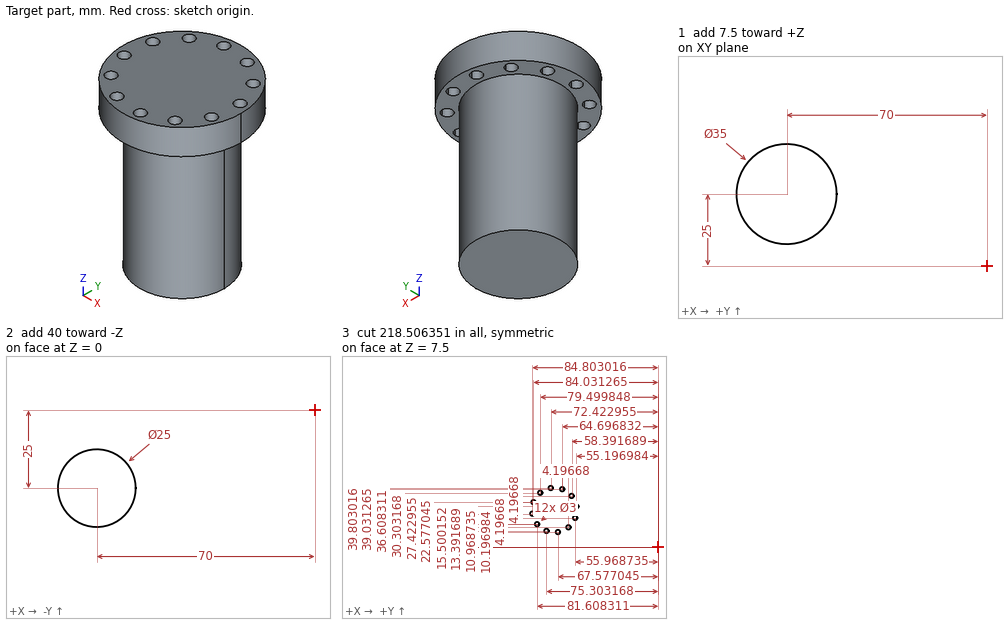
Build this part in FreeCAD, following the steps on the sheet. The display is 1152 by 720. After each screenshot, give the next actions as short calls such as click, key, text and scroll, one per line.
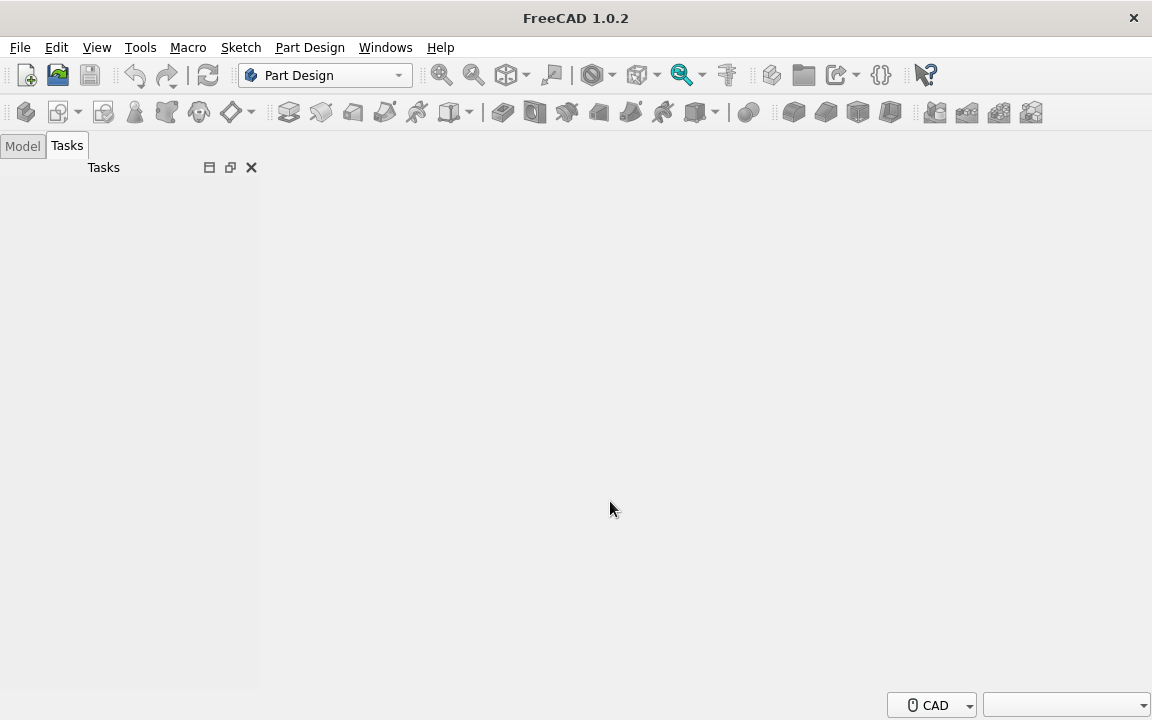
key(ctrl+n)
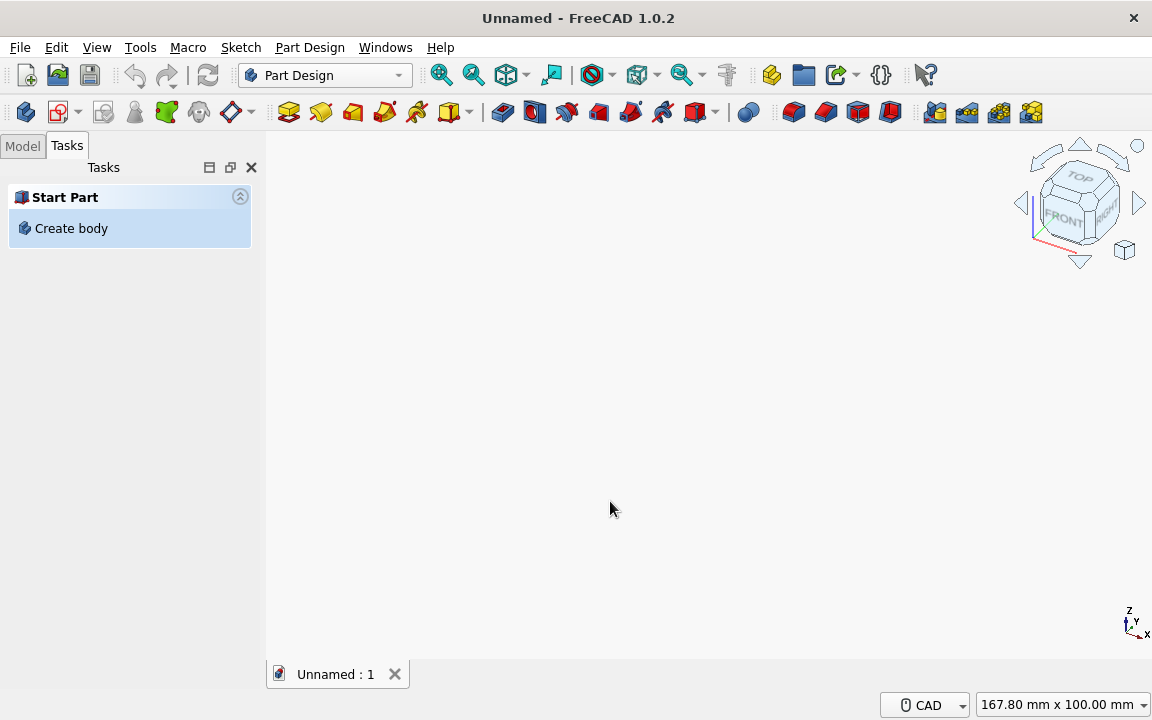
click(58, 112)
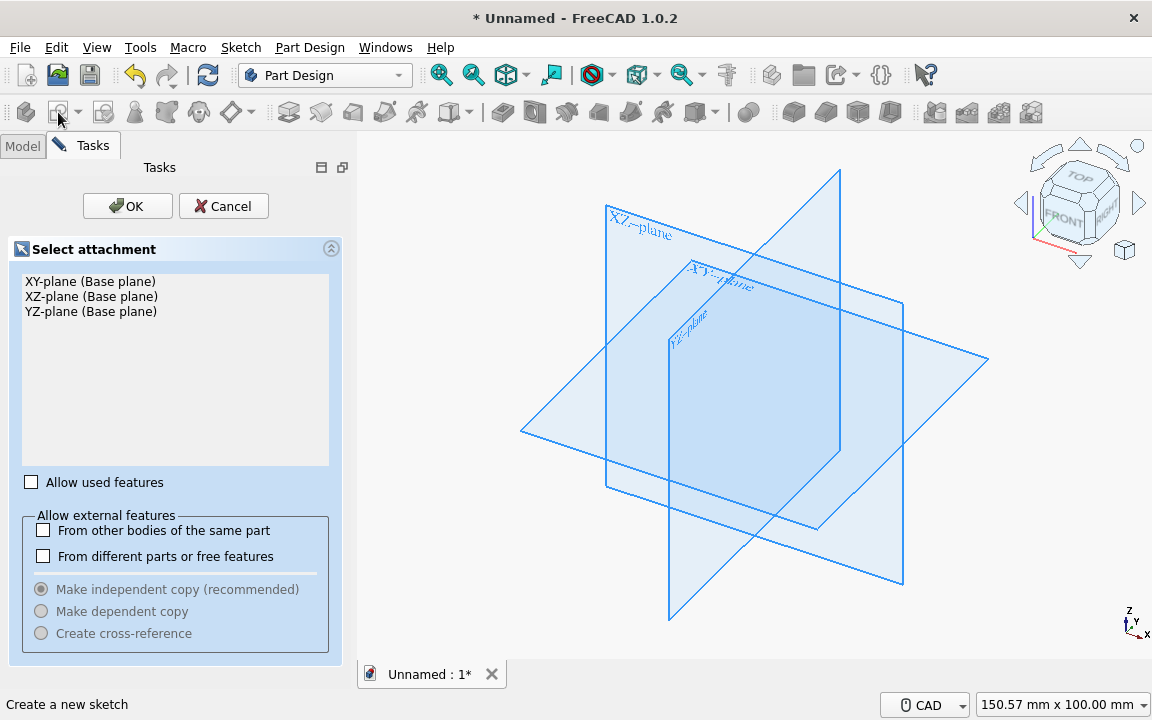
click(82, 282)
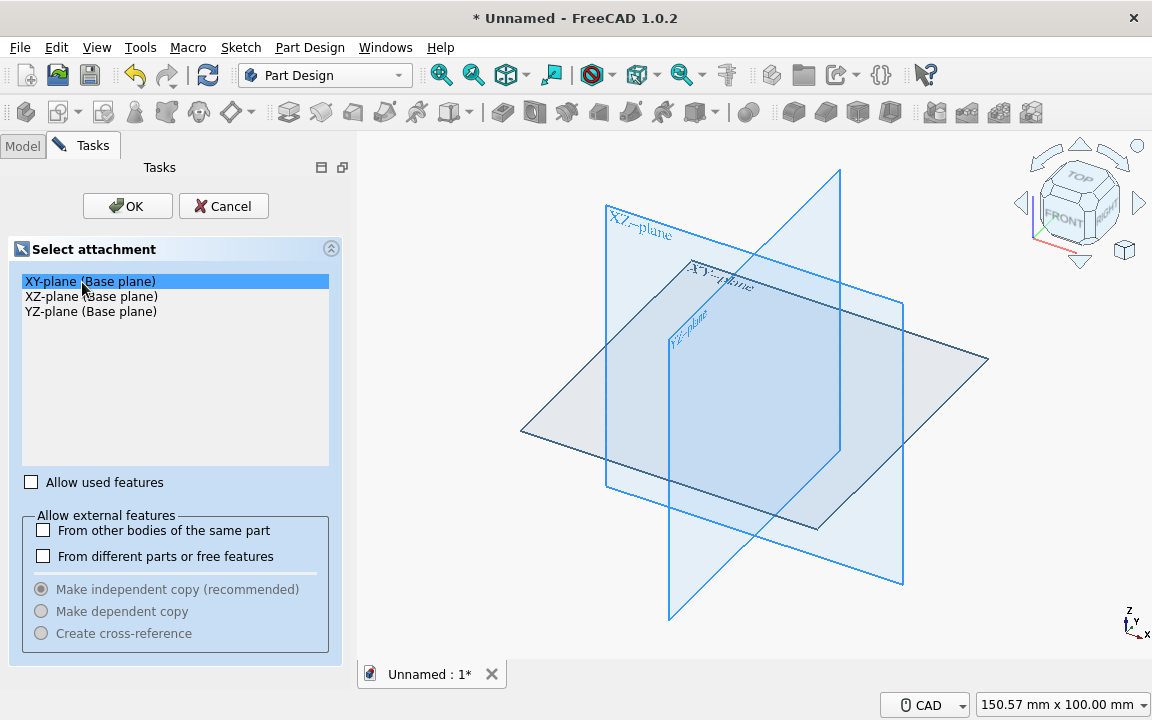
click(128, 206)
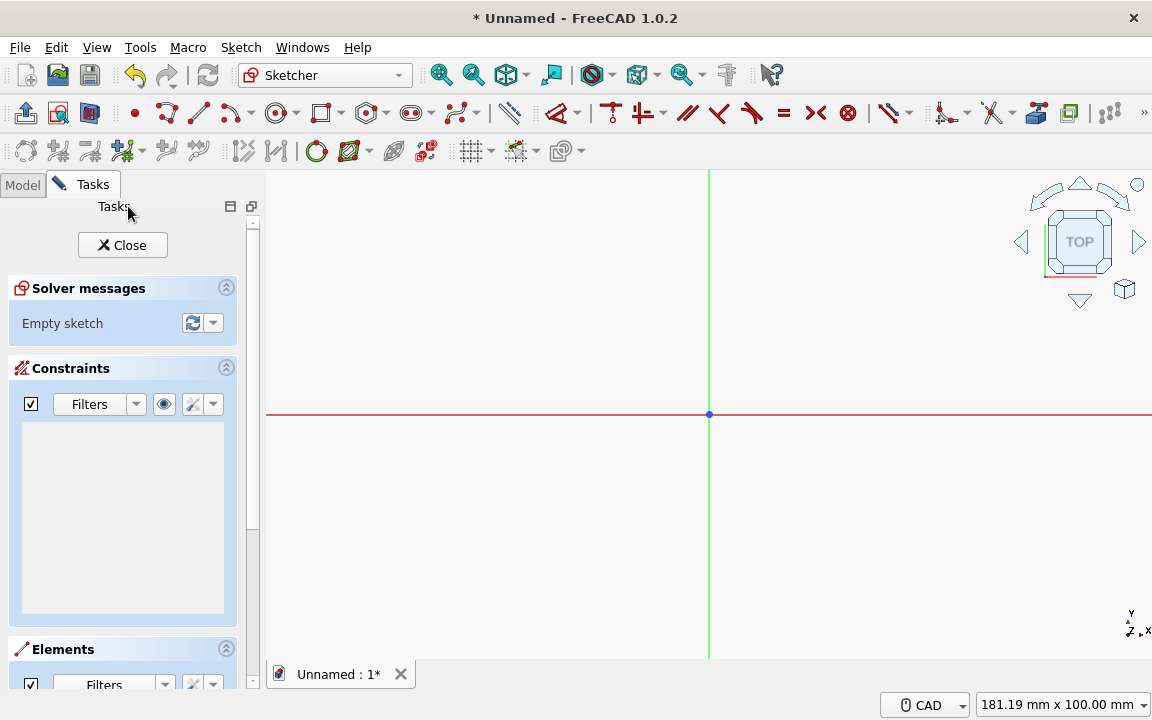
scroll(640, 414, down, 5)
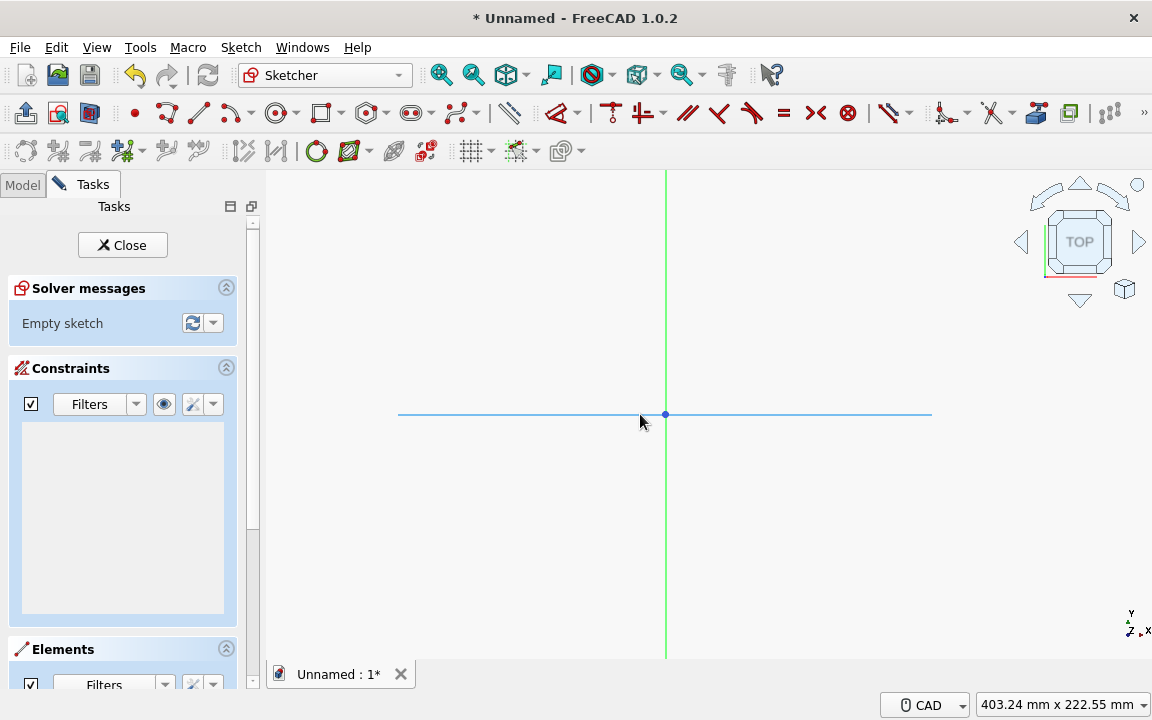
scroll(514, 358, up, 8)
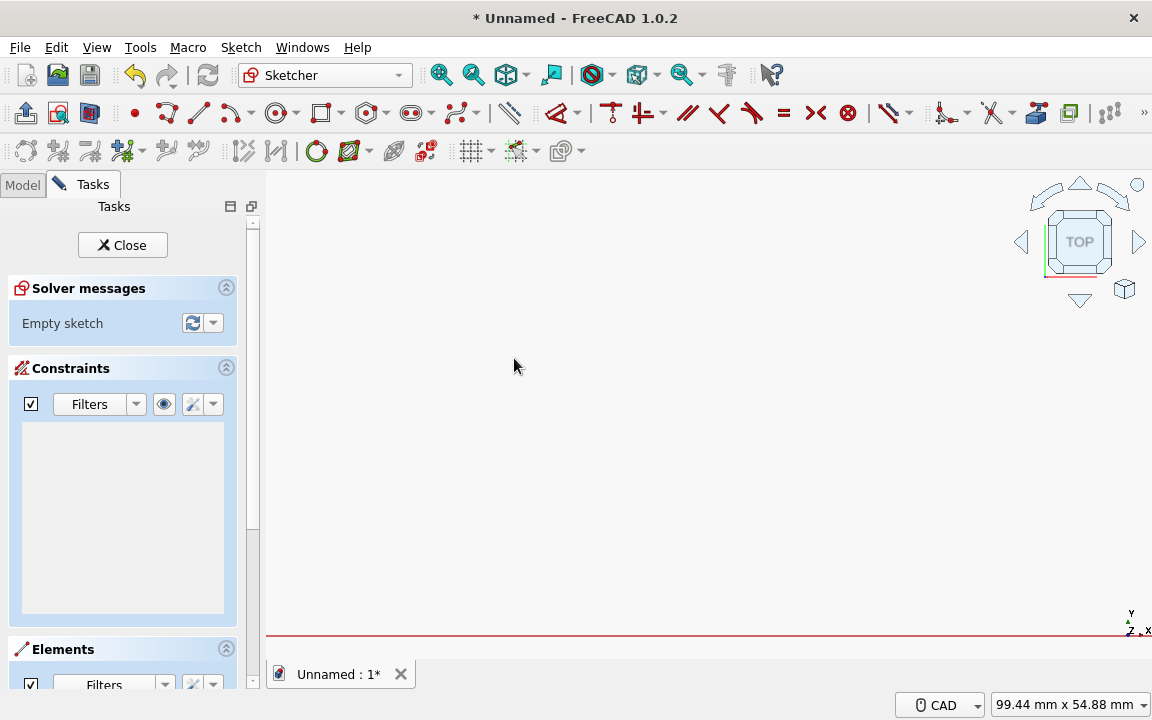
key(g)
key(c)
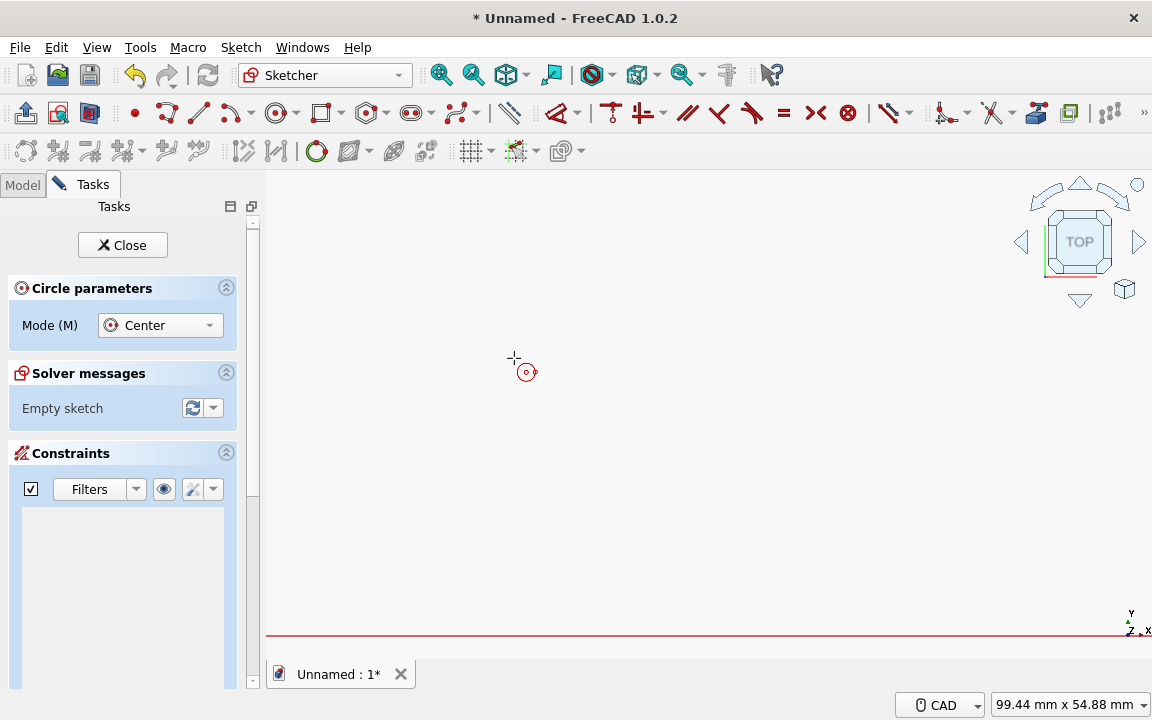
click(640, 414)
click(751, 303)
key(Escape)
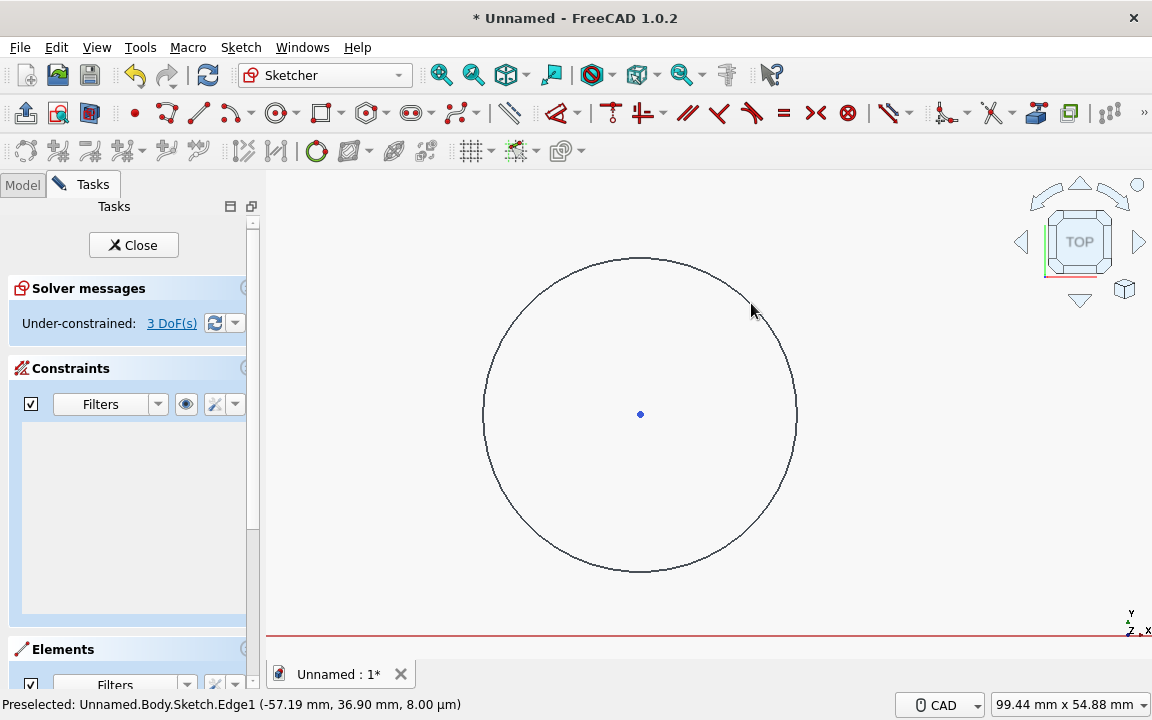
key(d)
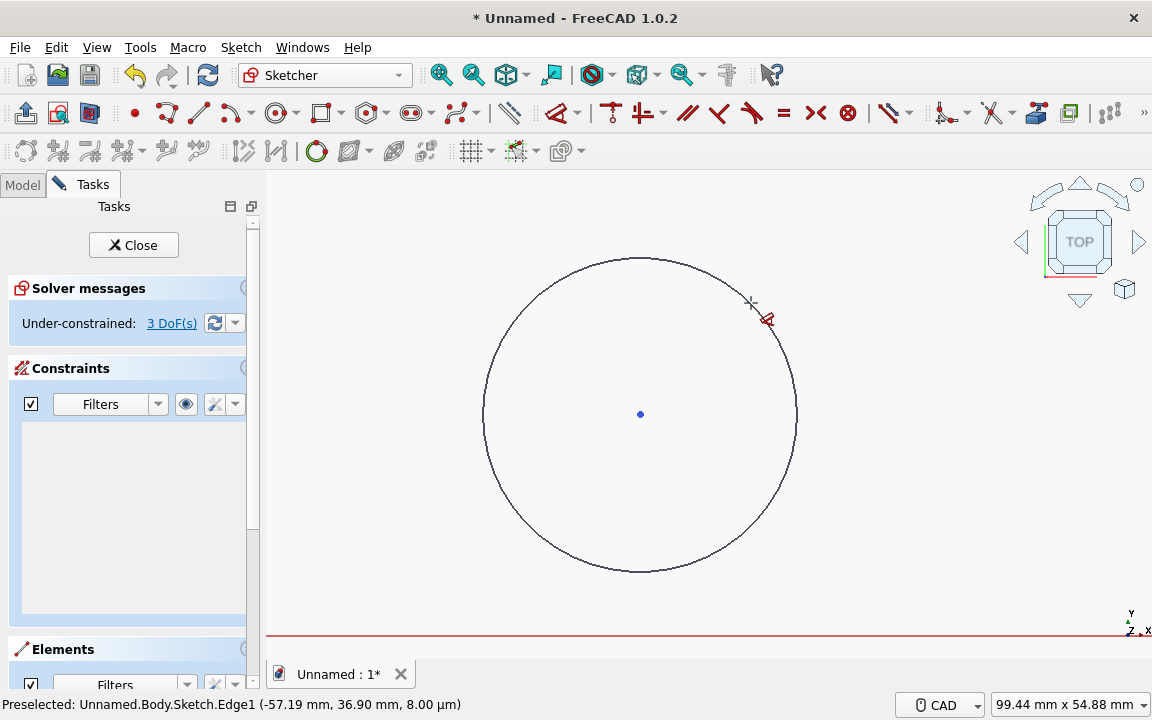
click(751, 304)
click(774, 281)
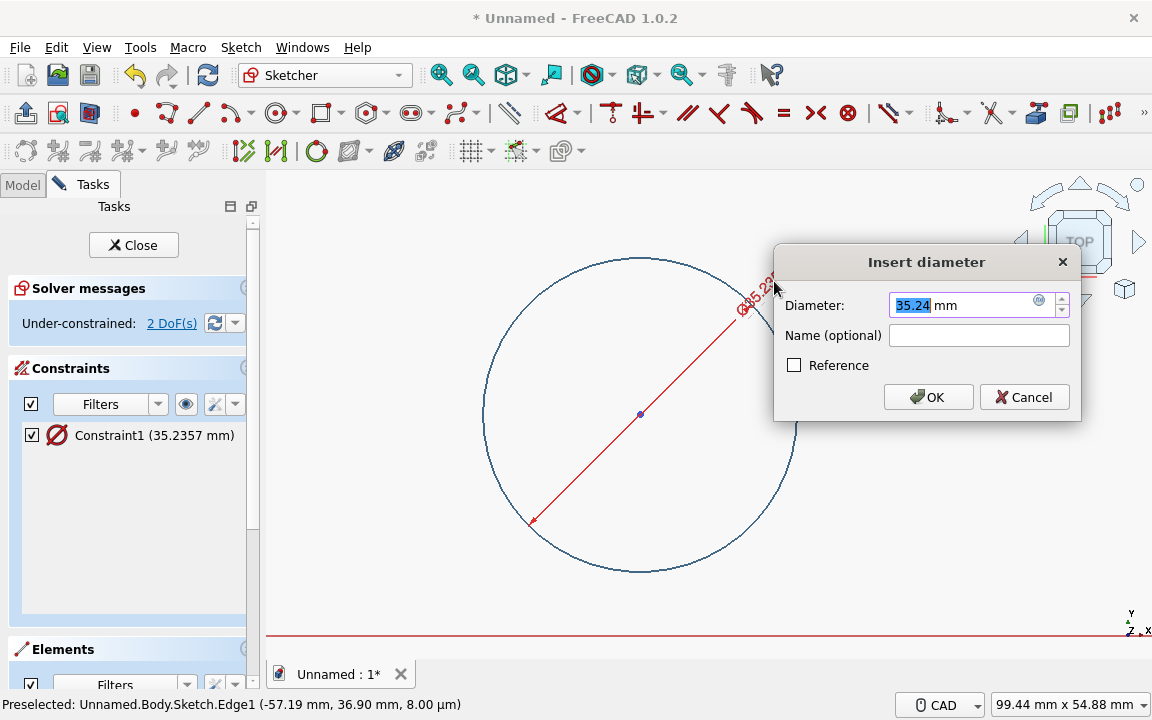
text(35)
key(Return)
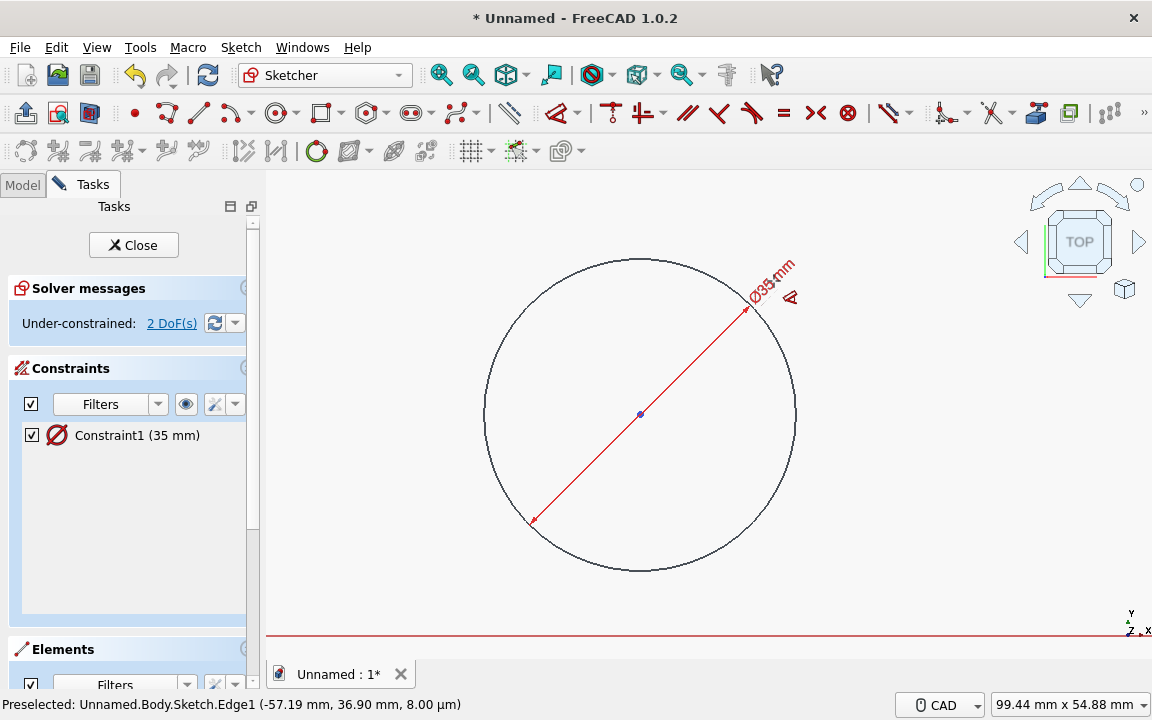
click(640, 415)
click(814, 381)